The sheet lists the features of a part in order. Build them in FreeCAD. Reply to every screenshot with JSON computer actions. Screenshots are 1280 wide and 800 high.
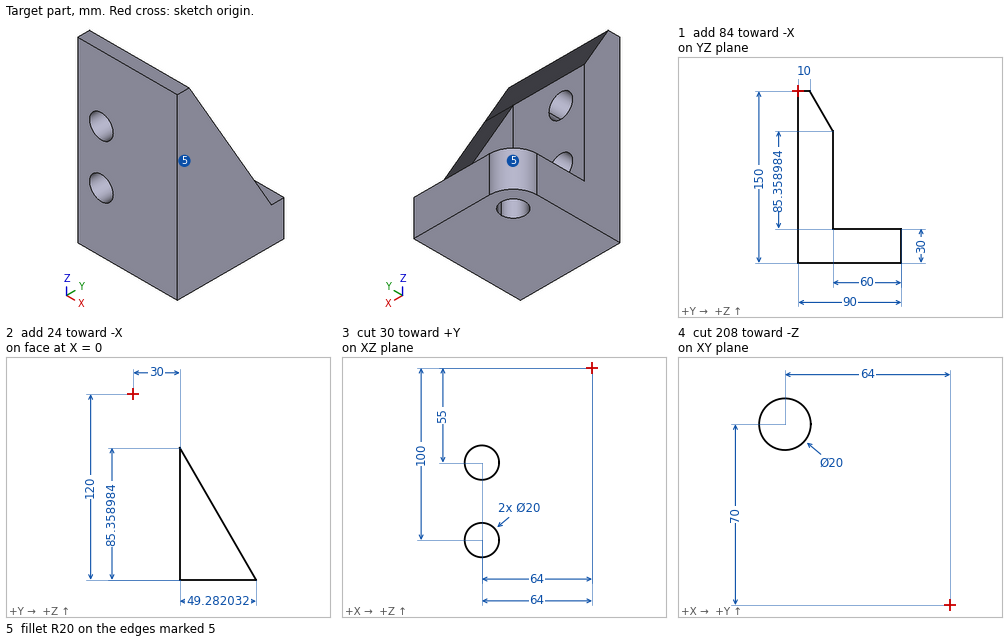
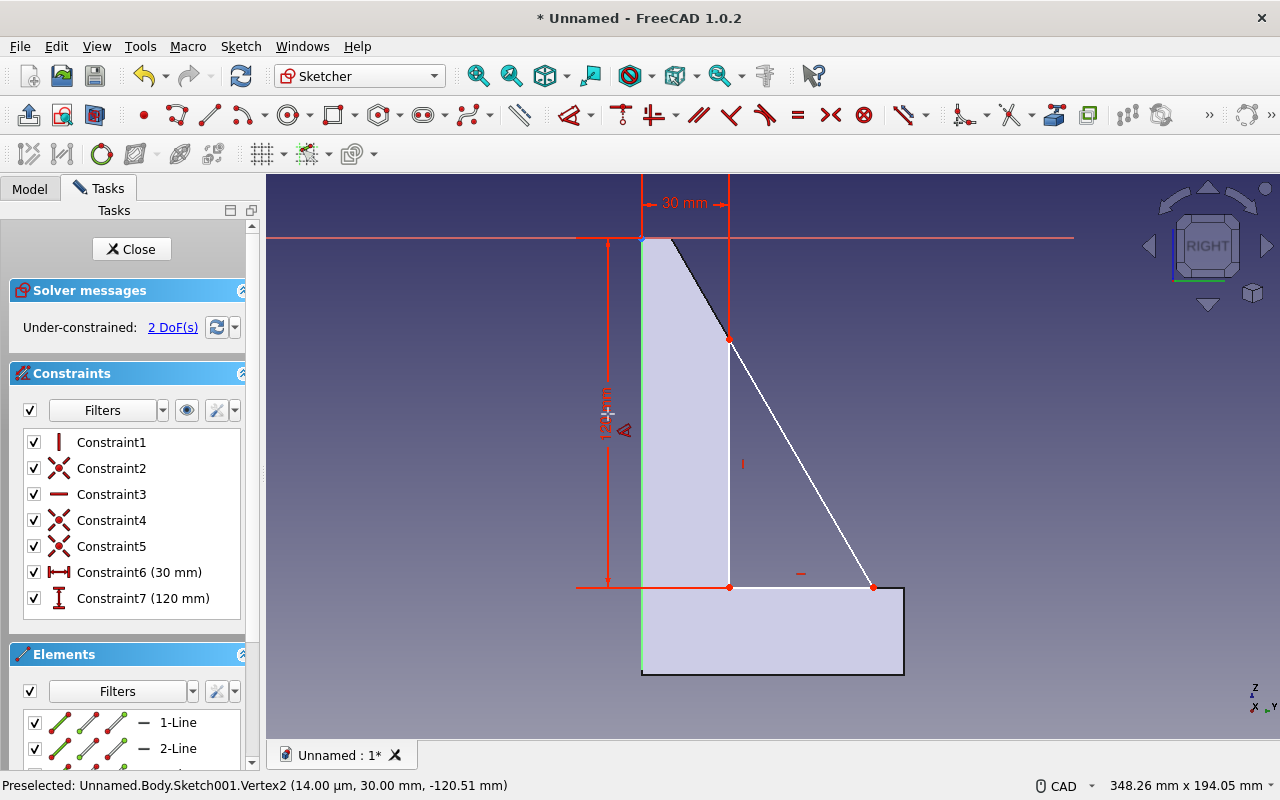
{"action": "left_click", "coordinate": [729, 414]}
{"action": "left_click", "coordinate": [695, 464]}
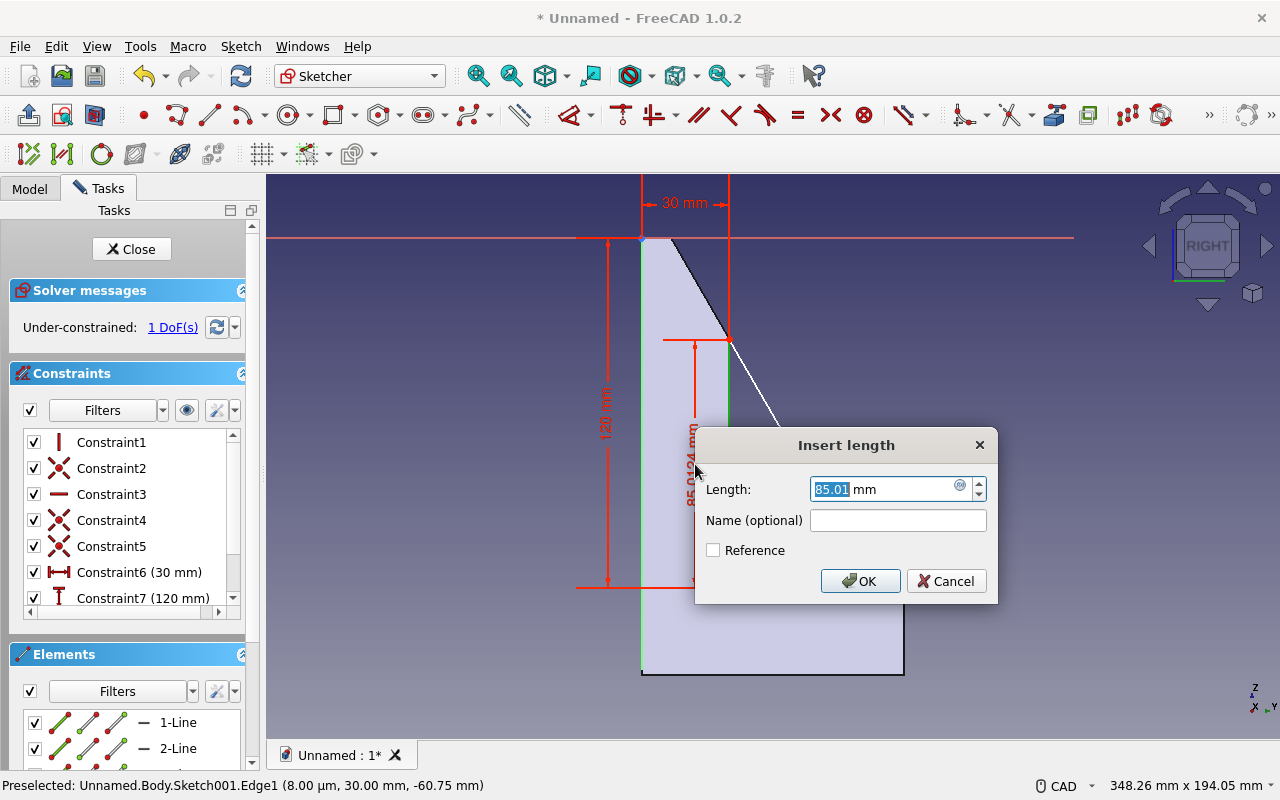
{"action": "type", "text": "85.358984"}
{"action": "key", "text": "Return"}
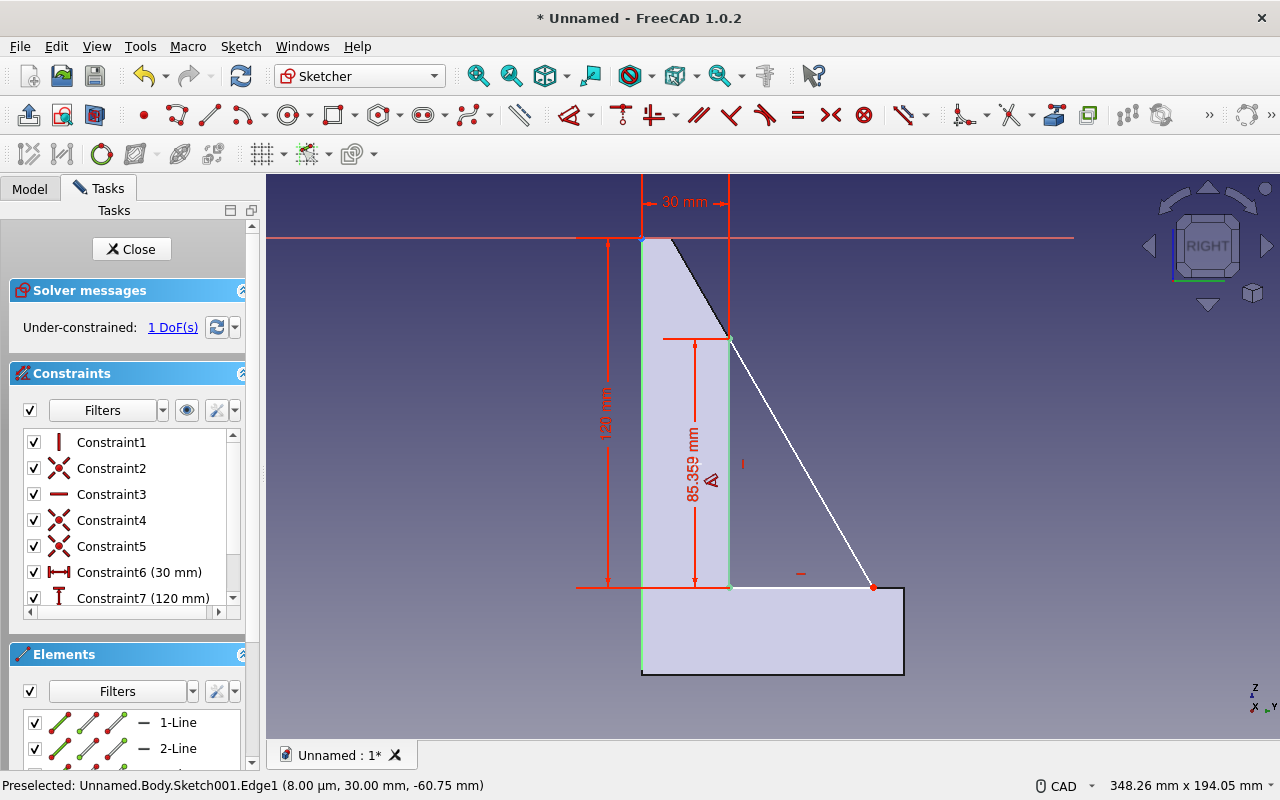
{"action": "left_click", "coordinate": [772, 588]}
{"action": "left_click", "coordinate": [801, 622]}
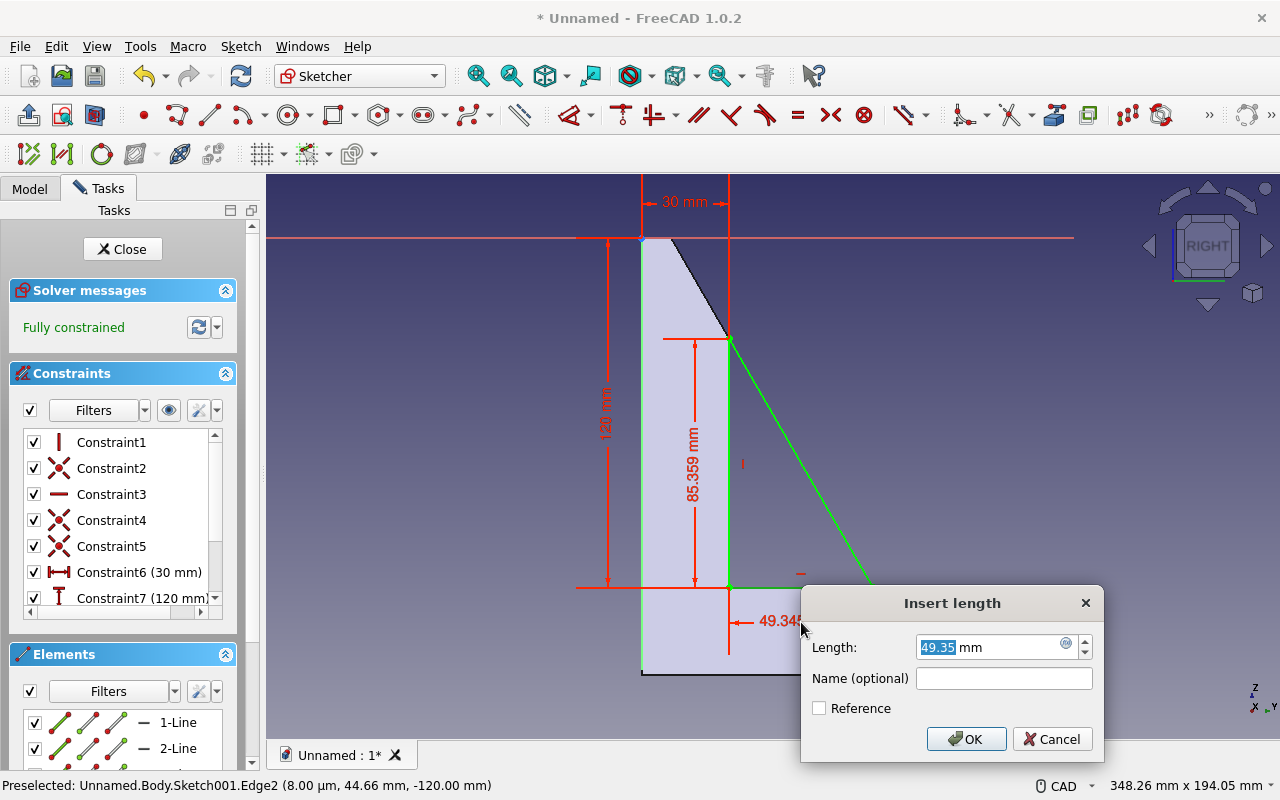
{"action": "type", "text": "49.282032"}
{"action": "key", "text": "Return"}
{"action": "key", "text": "Escape"}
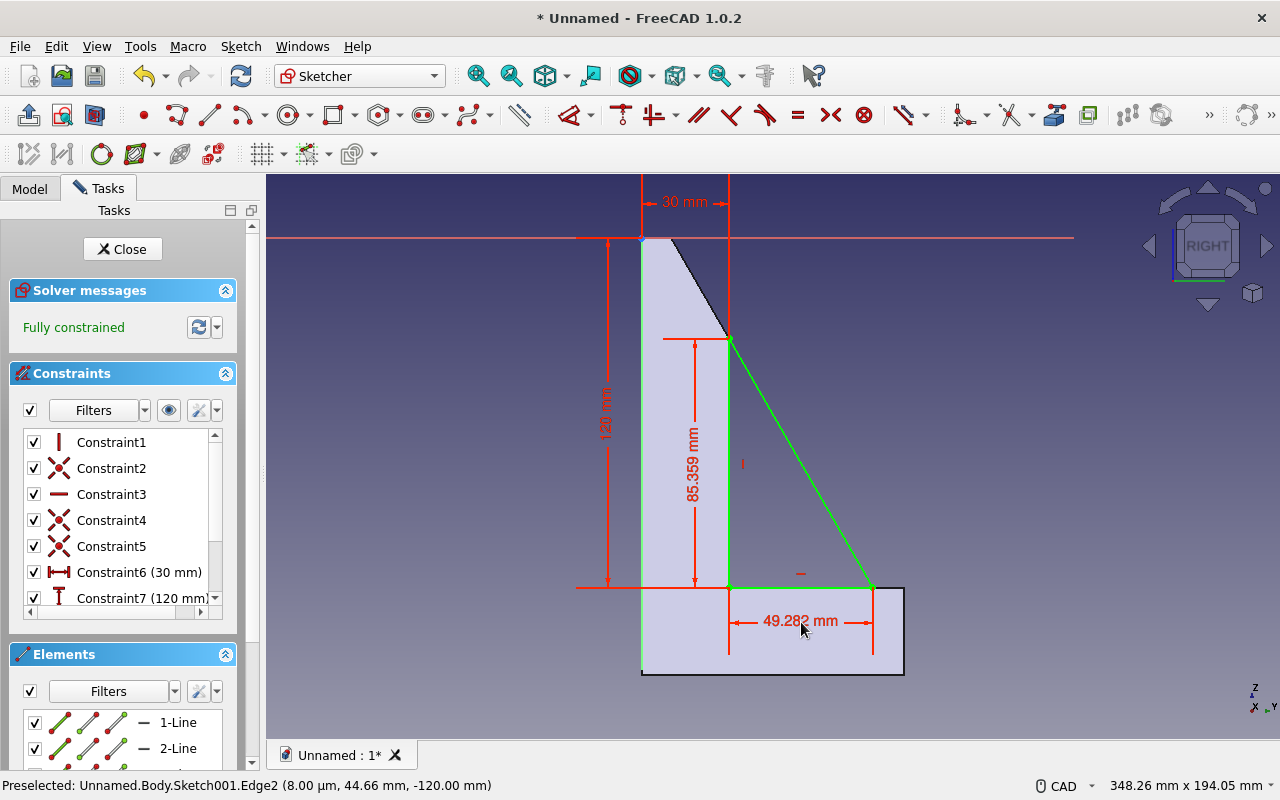
{"action": "left_click", "coordinate": [123, 249]}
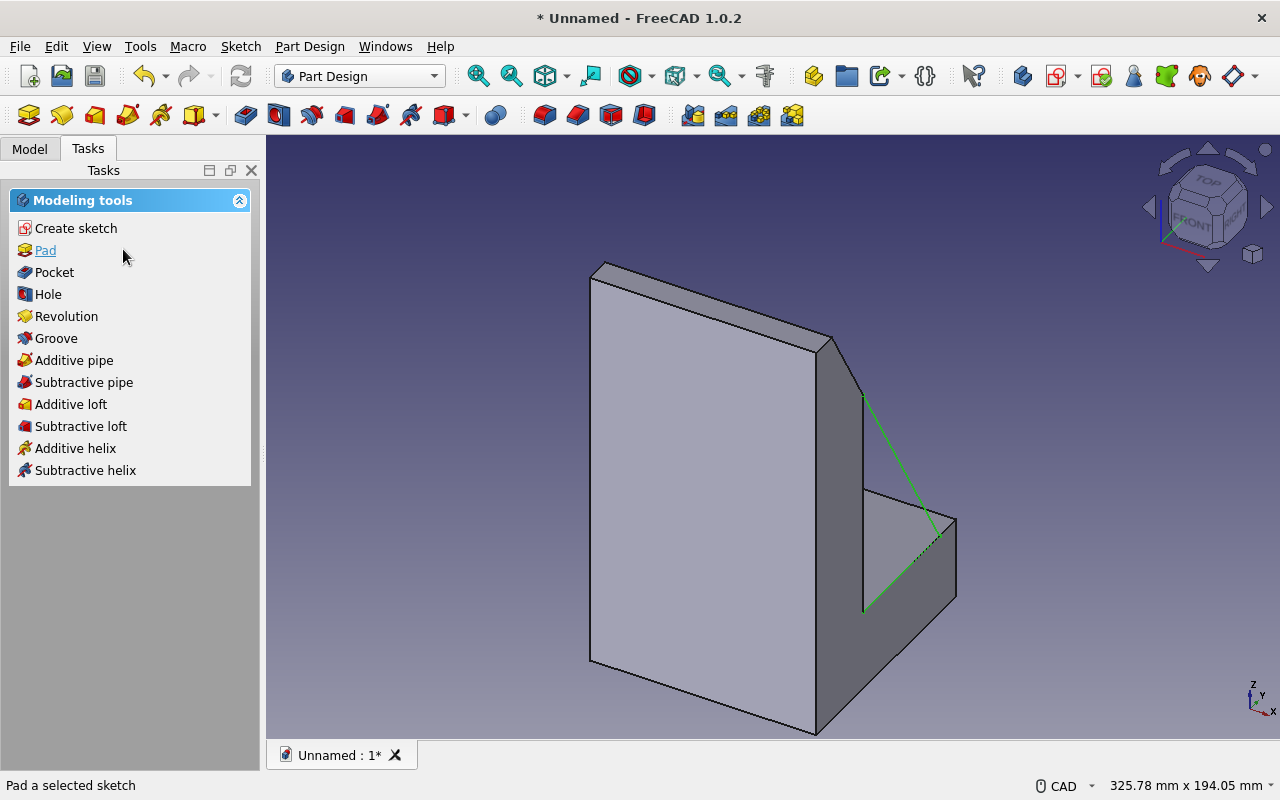
{"action": "left_click", "coordinate": [29, 116]}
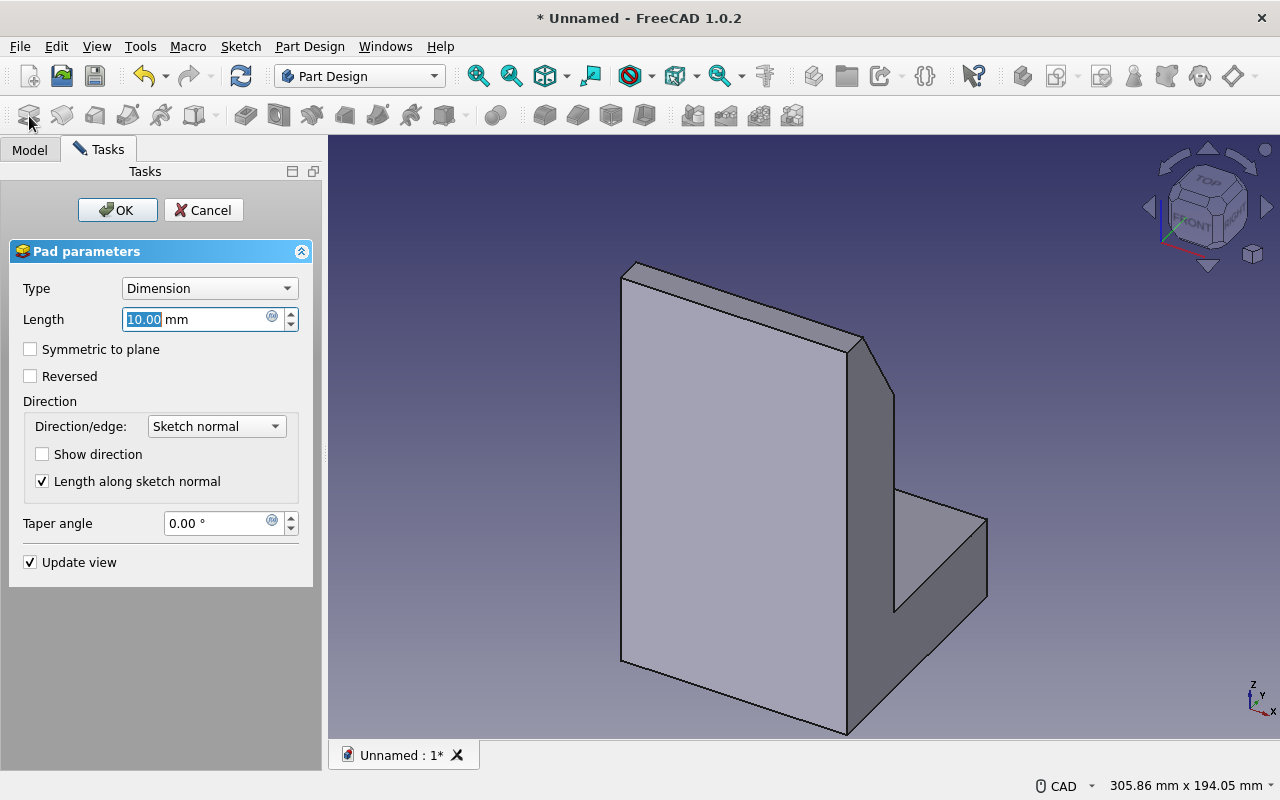
{"action": "type", "text": "24"}
{"action": "key", "text": "Tab"}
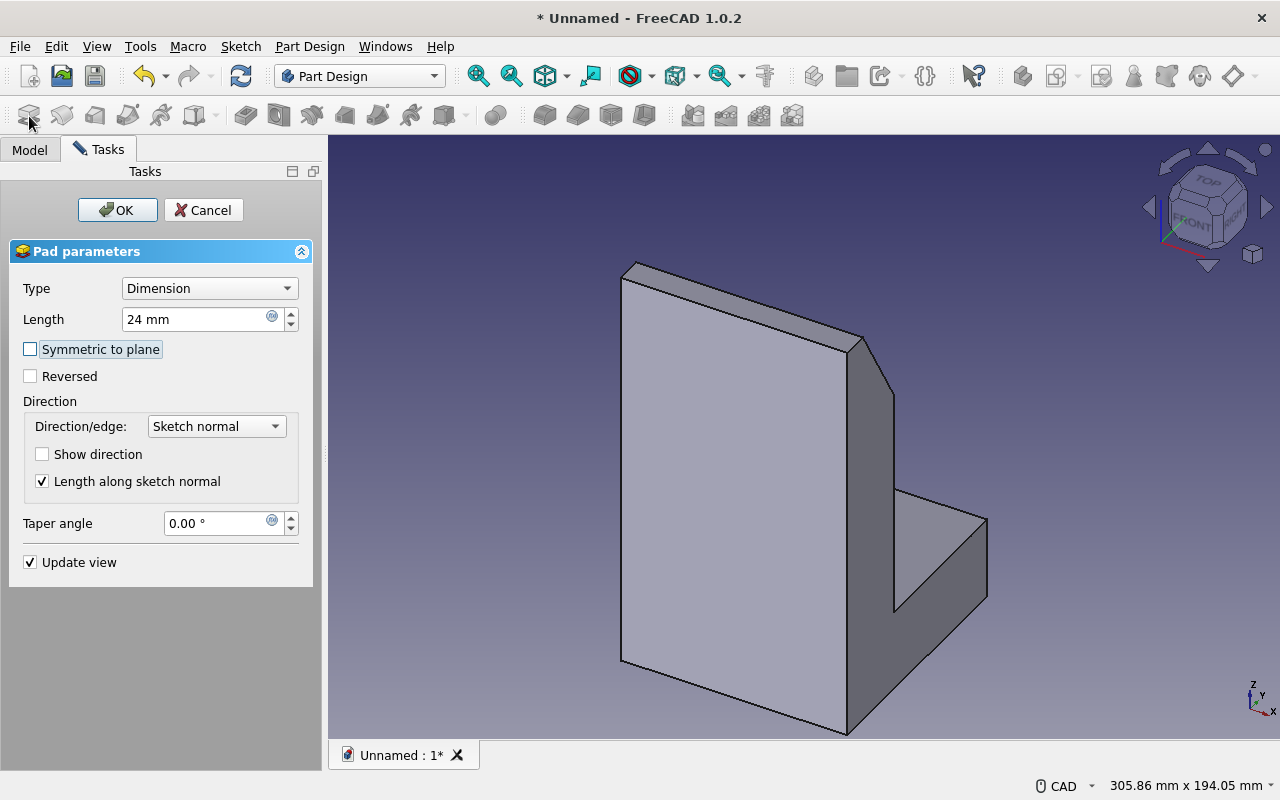
{"action": "left_click", "coordinate": [31, 376]}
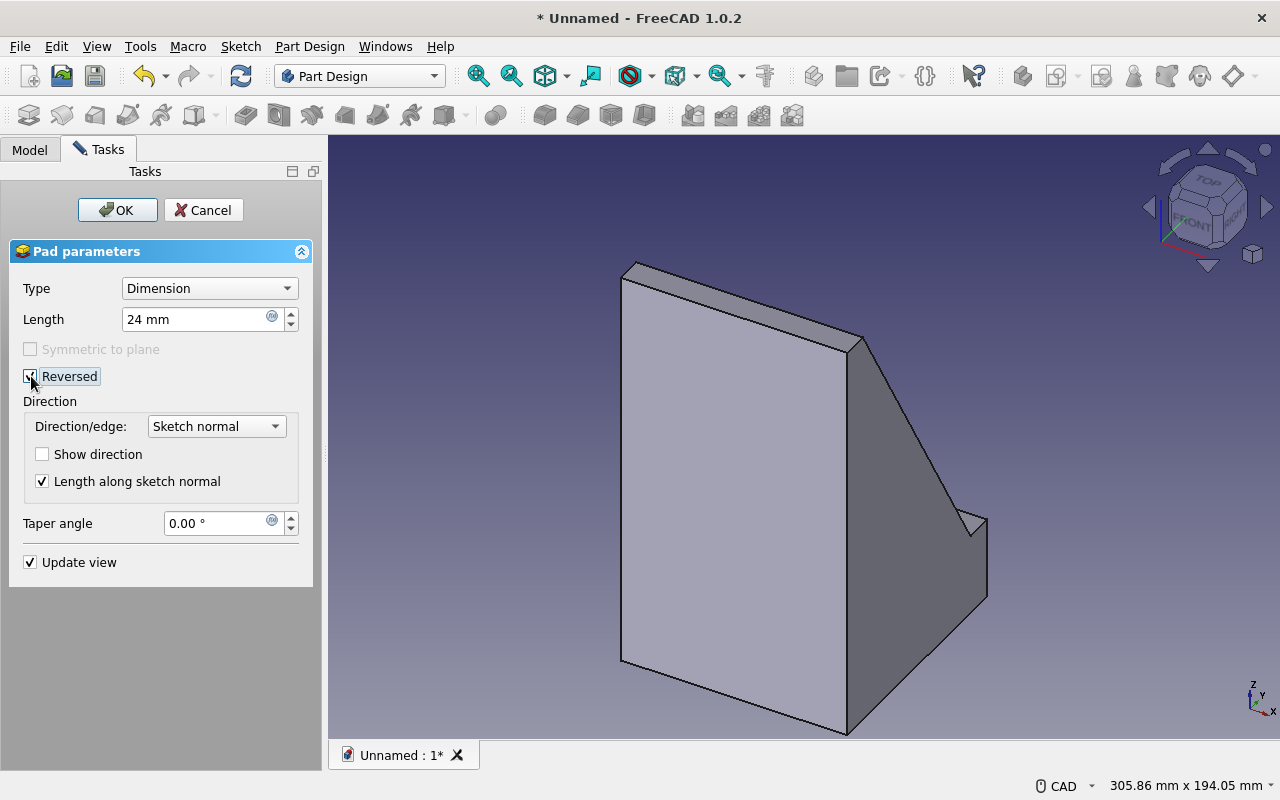
{"action": "left_click", "coordinate": [118, 210]}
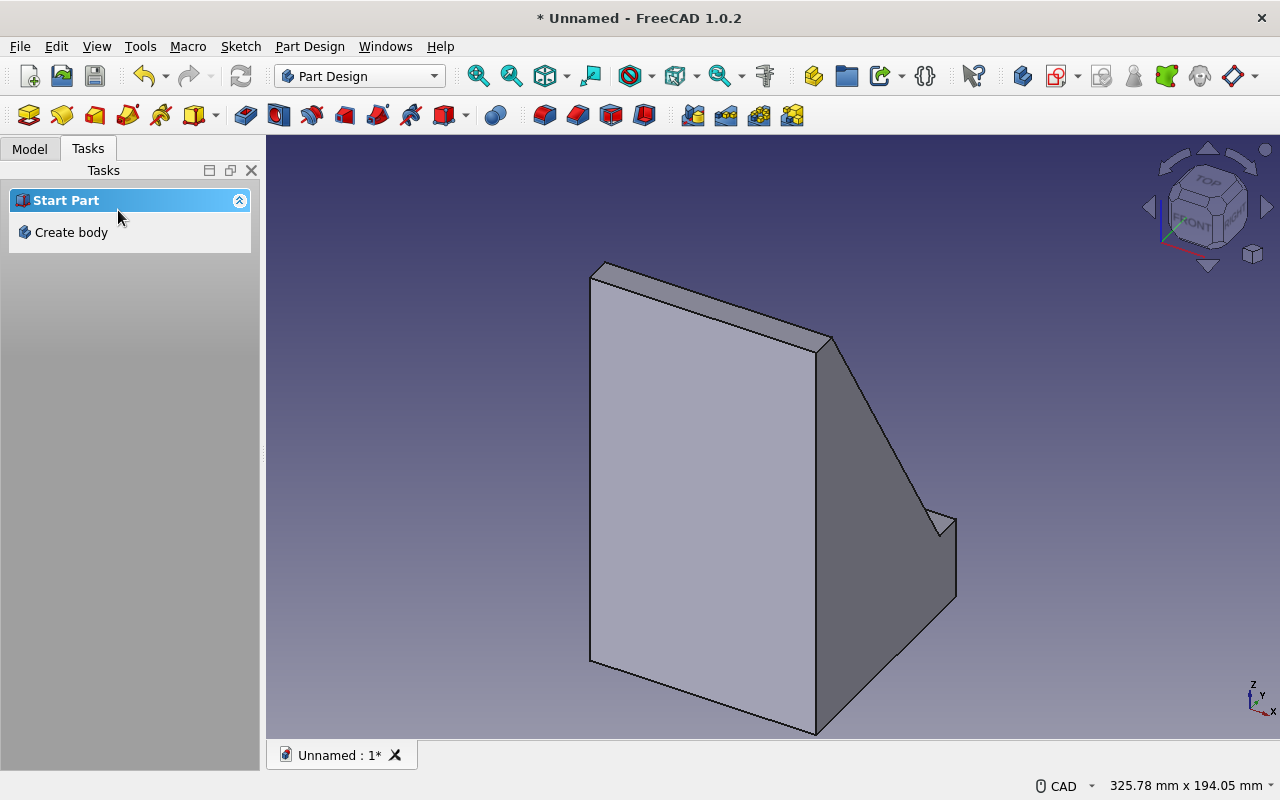
{"action": "left_click", "coordinate": [1056, 76]}